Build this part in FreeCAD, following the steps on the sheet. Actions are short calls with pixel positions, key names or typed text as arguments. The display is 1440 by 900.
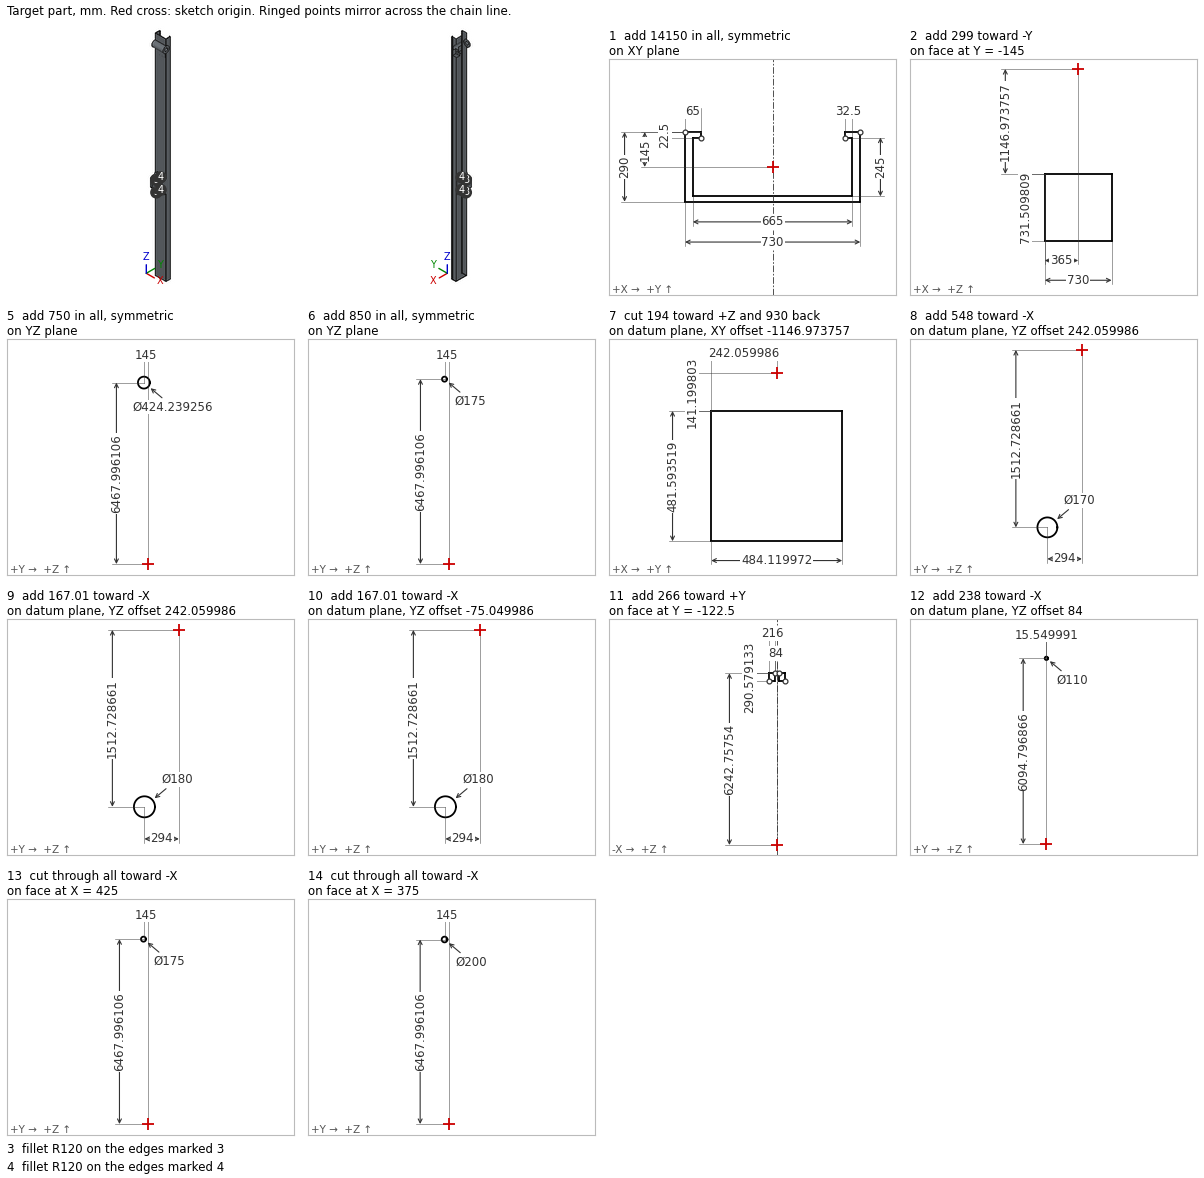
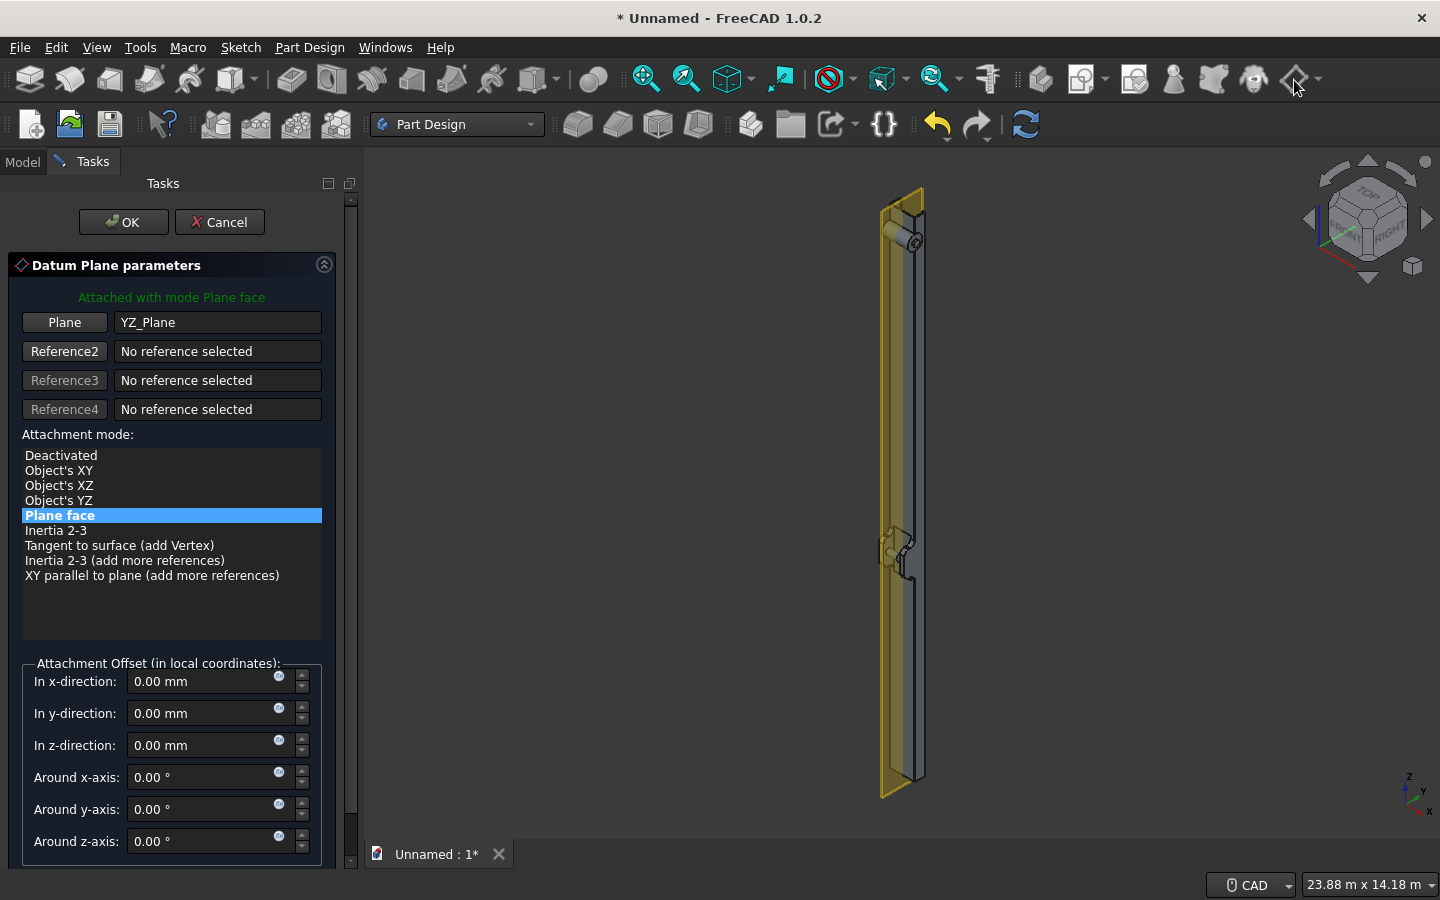
triple_click(210, 745)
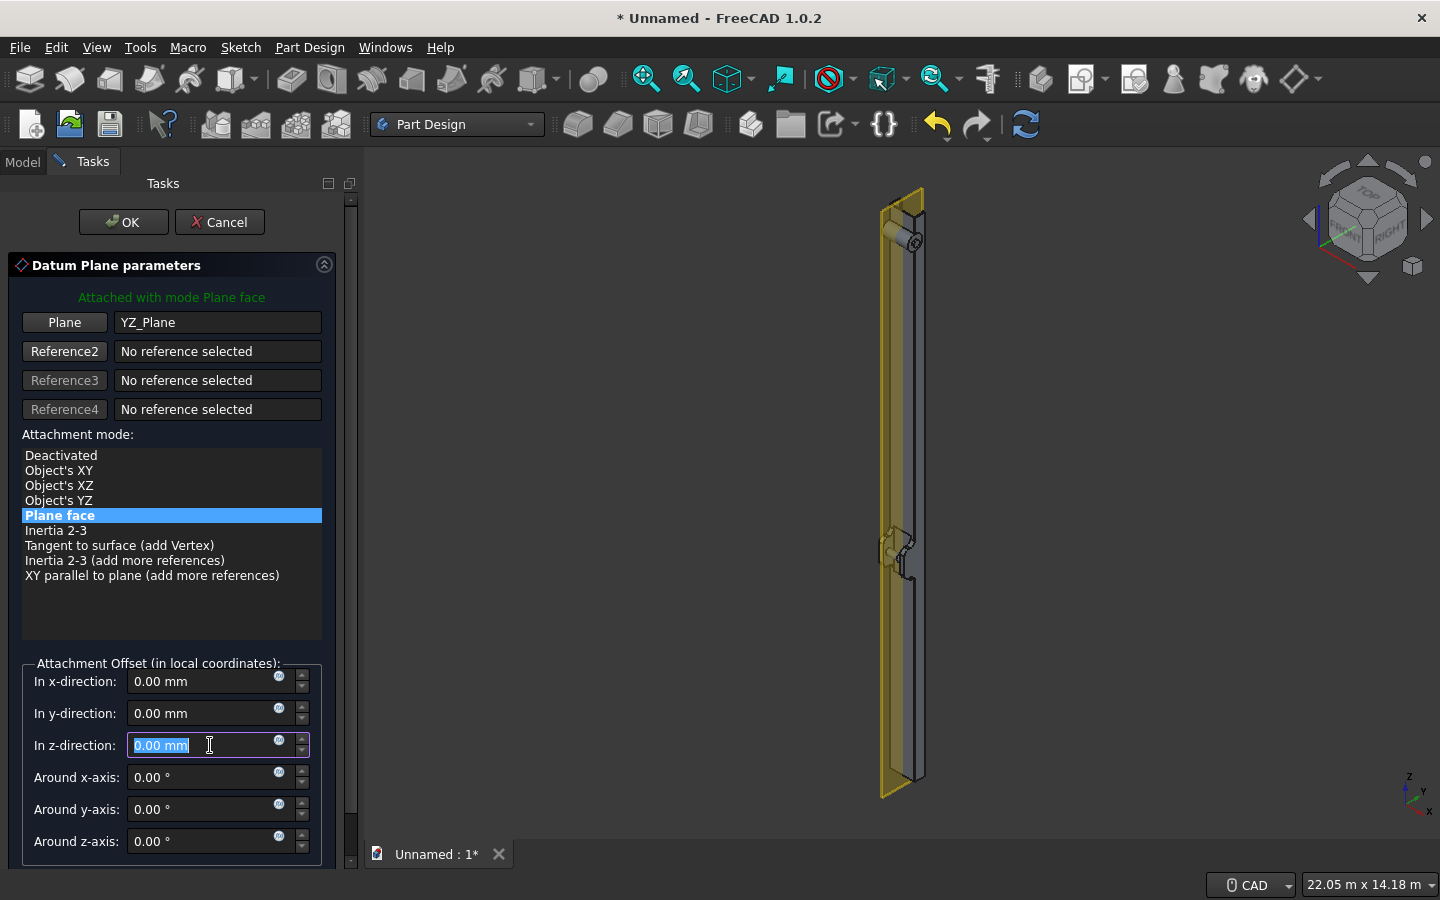
text(-75.049986)
key(Tab)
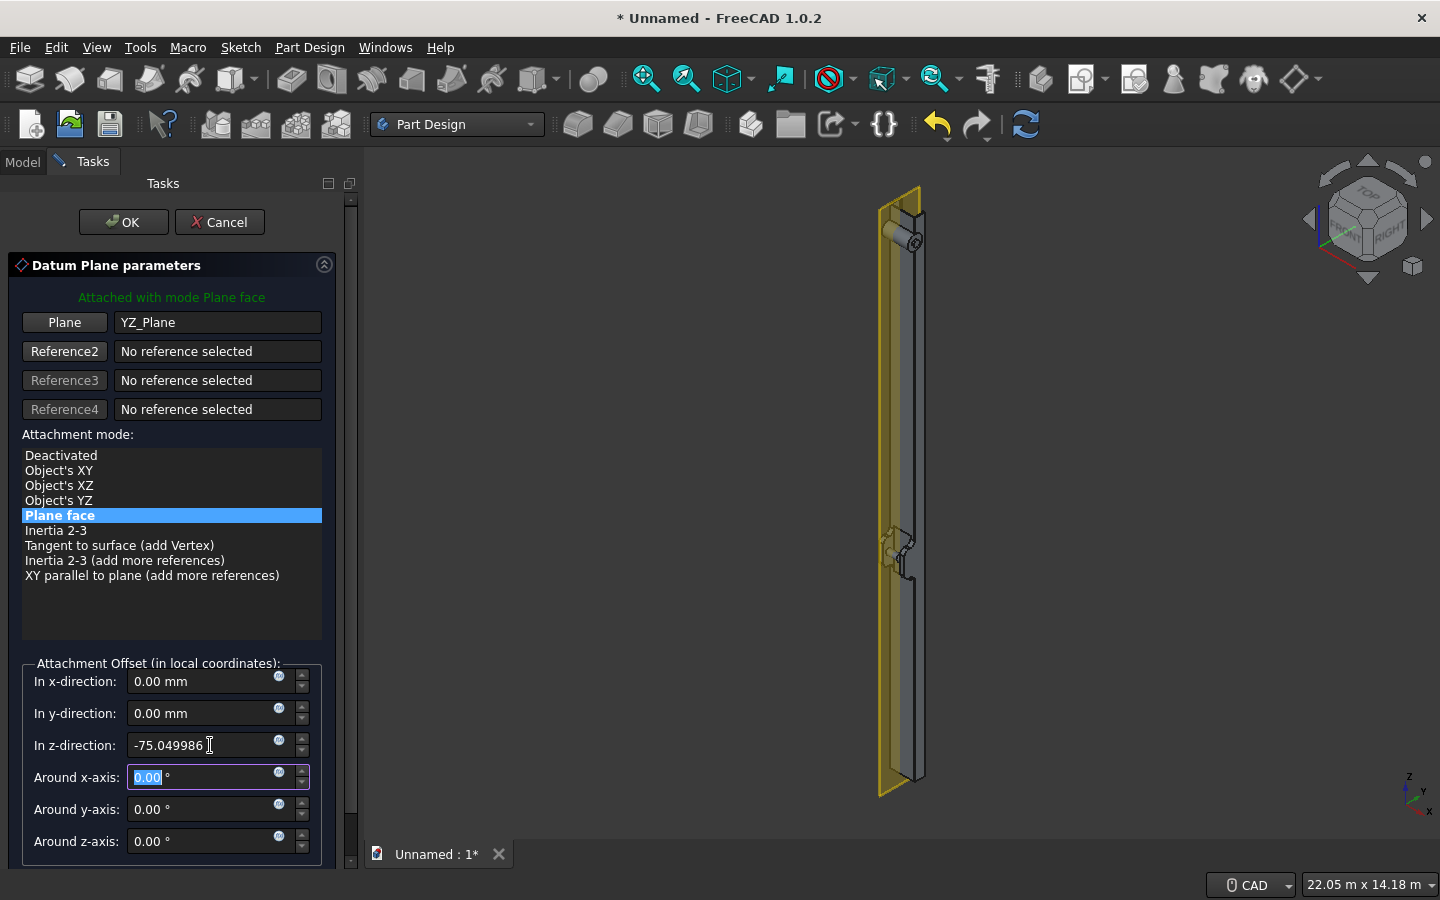
click(124, 222)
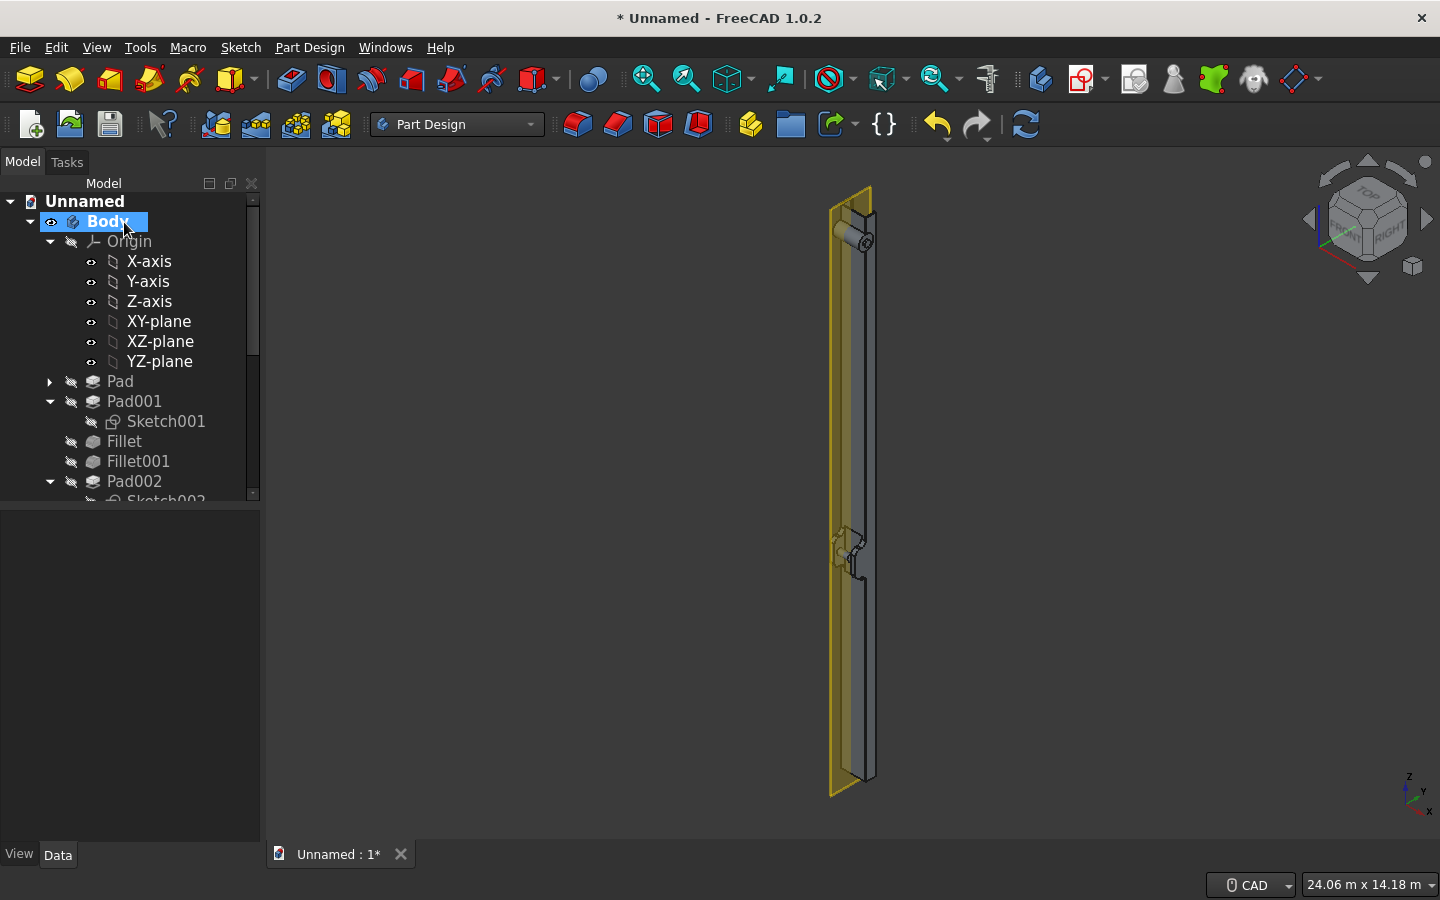
scroll(100, 337, down, 3)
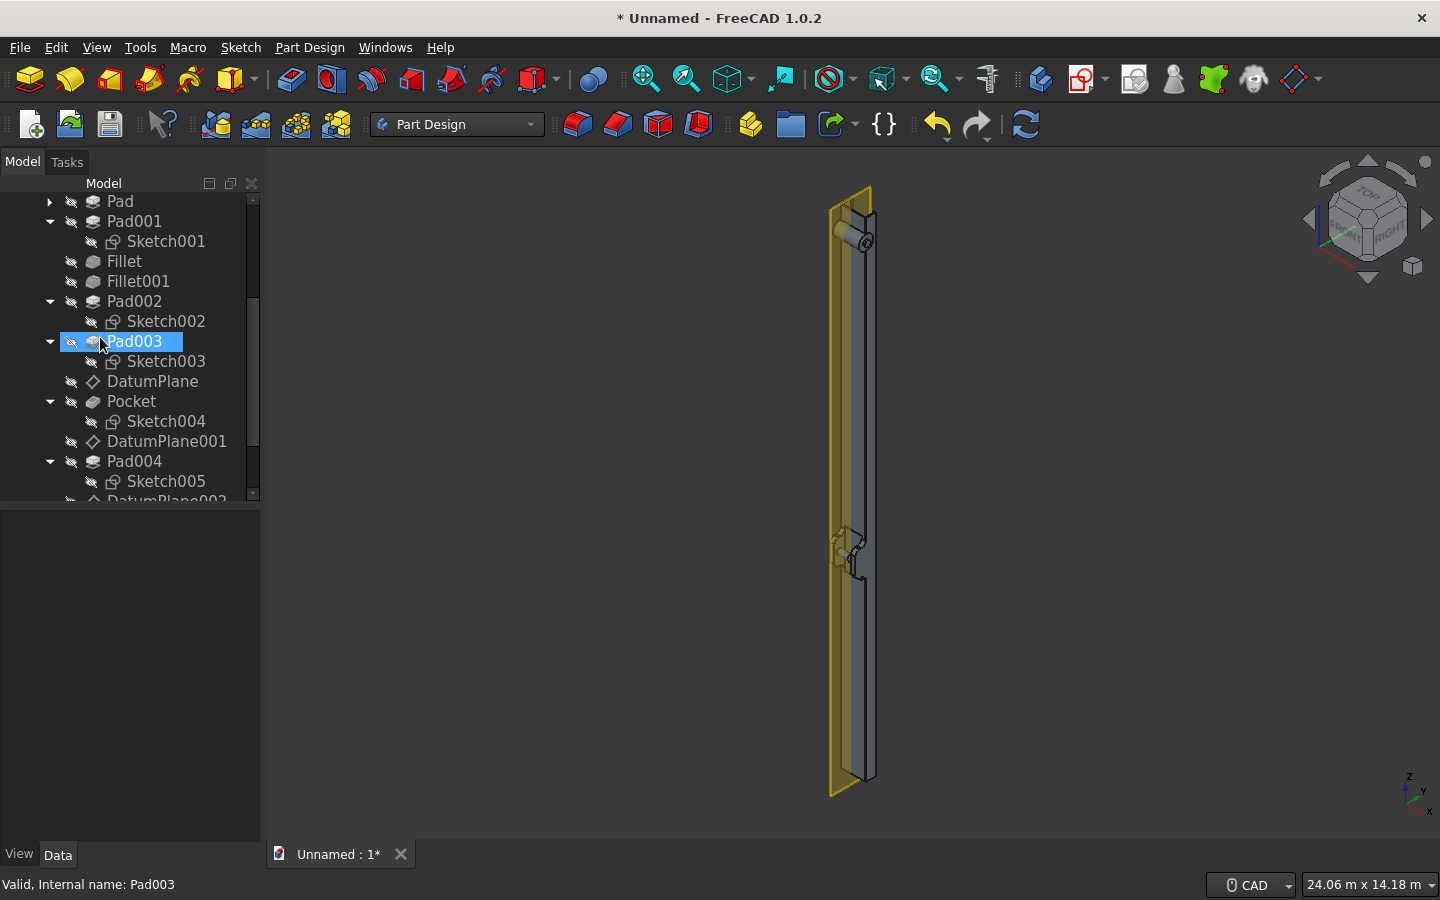
scroll(140, 337, up, 15)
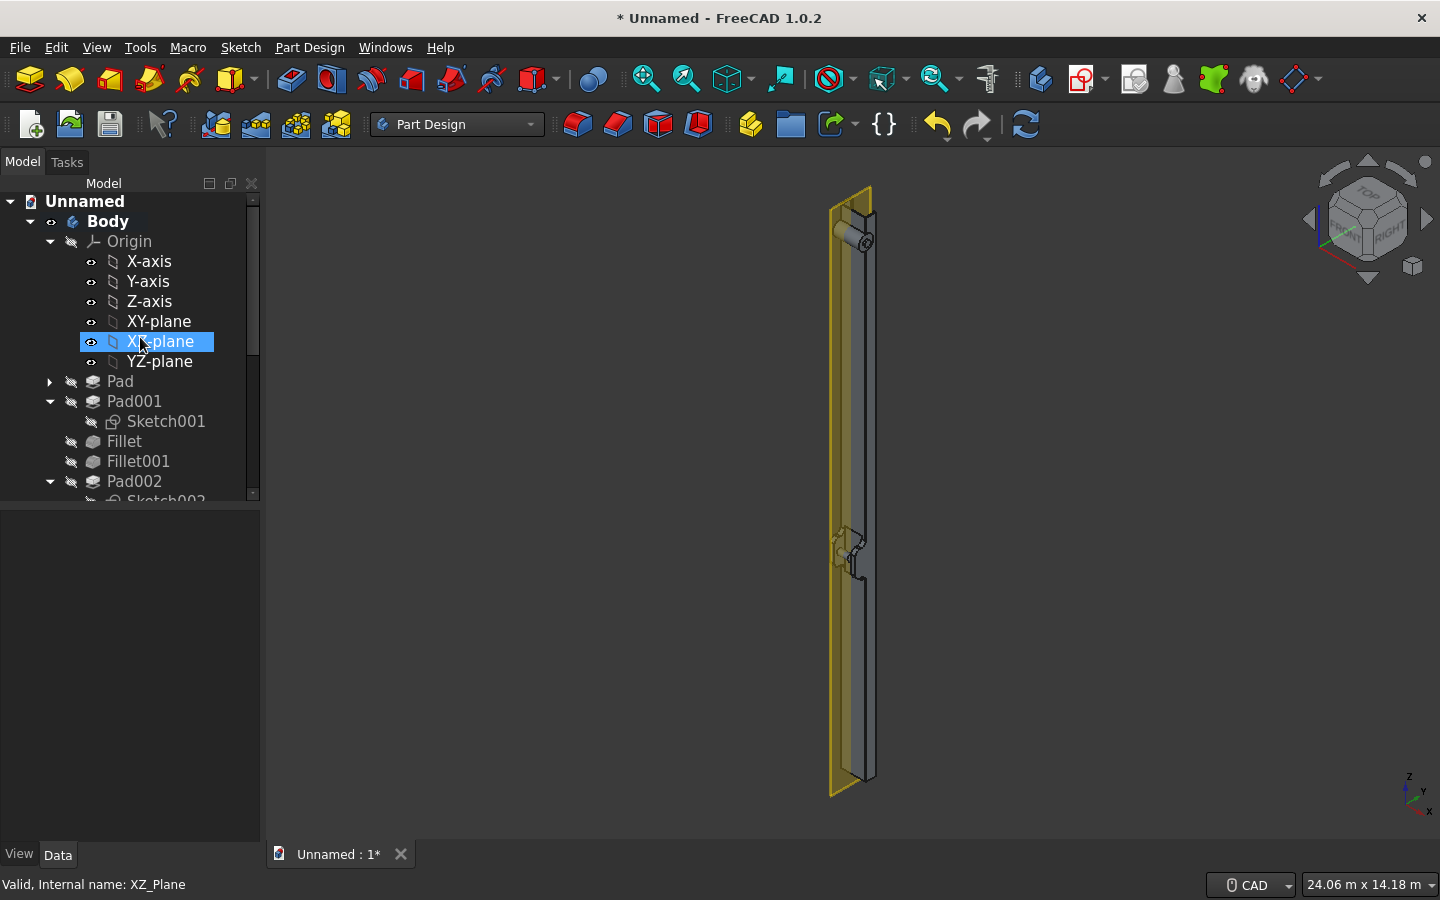
scroll(100, 337, down, 6)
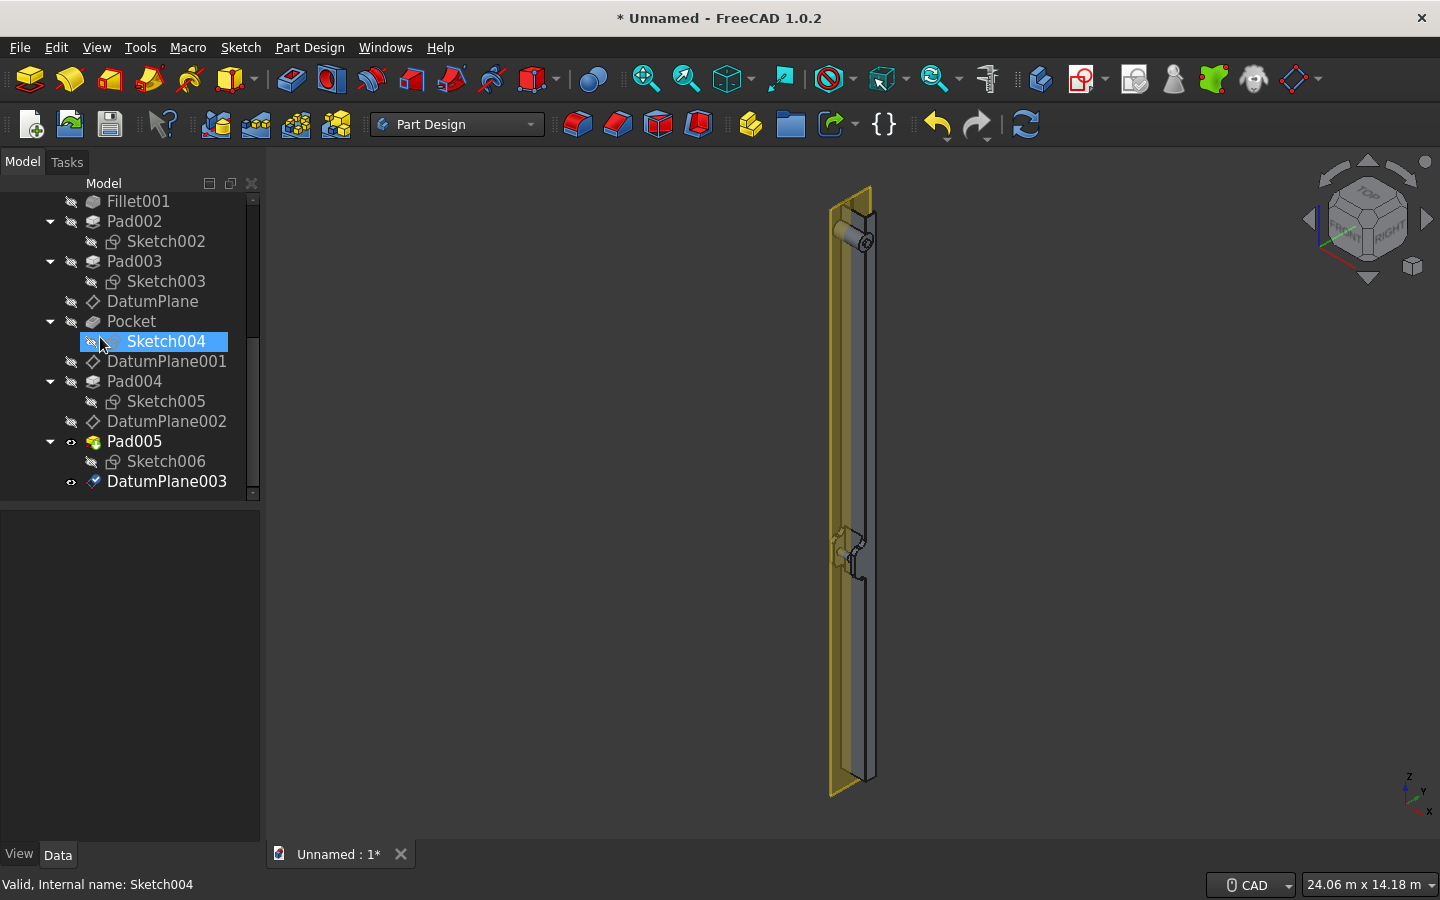
click(116, 482)